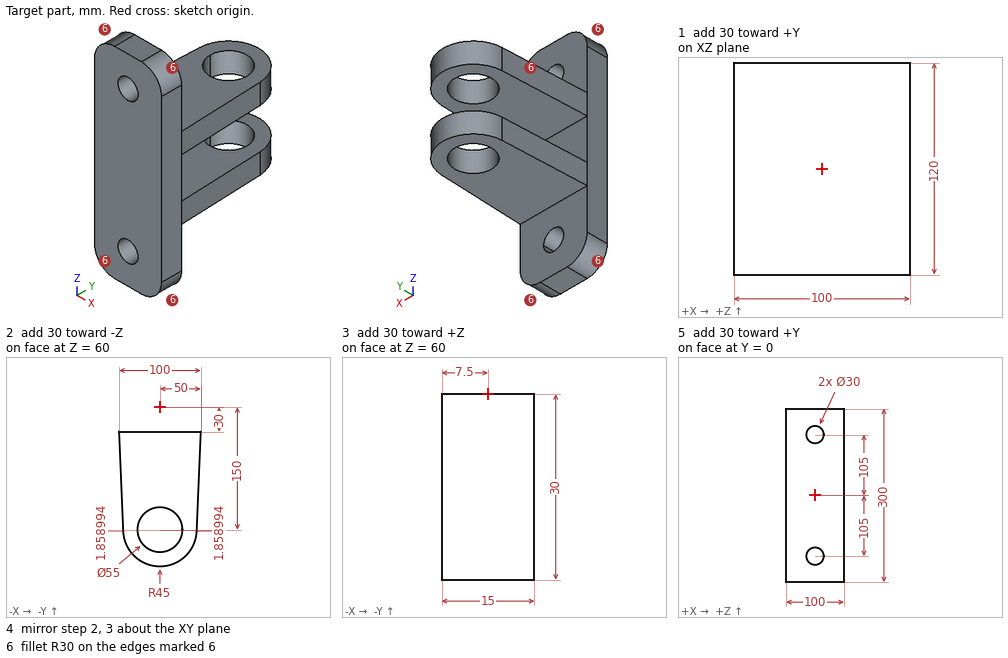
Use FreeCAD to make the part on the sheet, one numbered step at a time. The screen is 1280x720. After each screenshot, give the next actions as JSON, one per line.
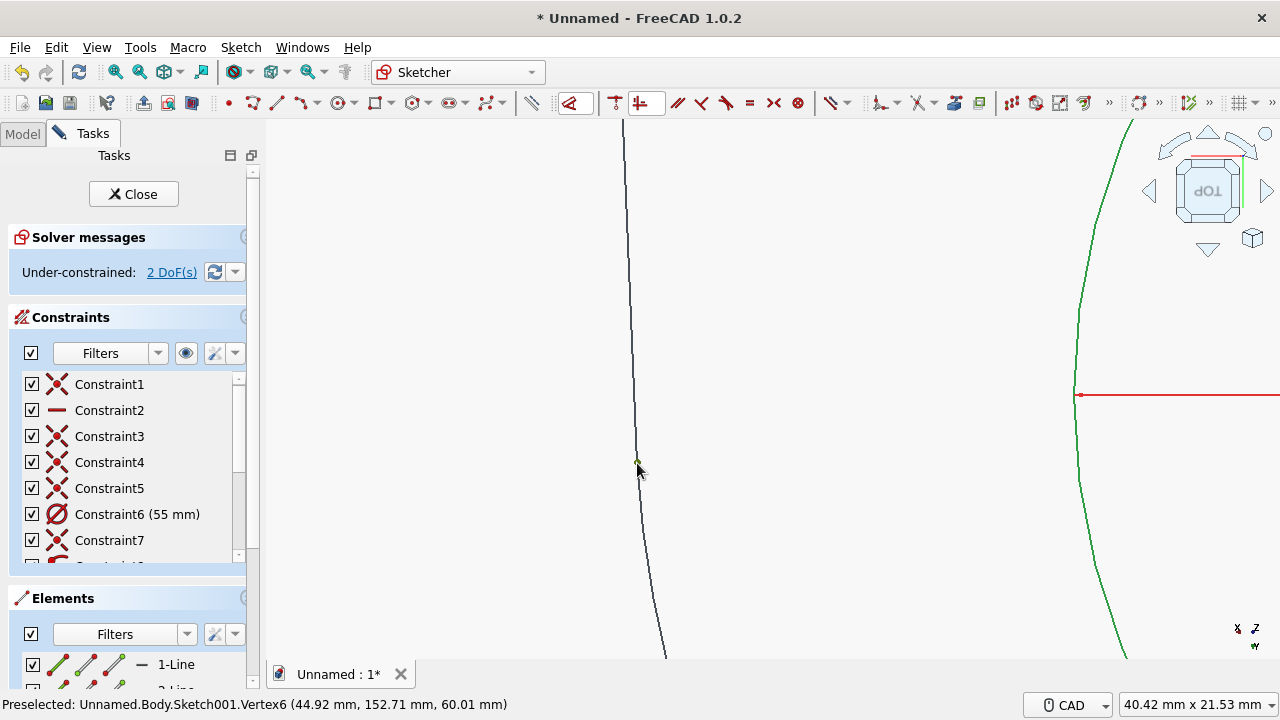
{"action": "scroll", "coordinate": [620, 494], "scroll_direction": "down", "scroll_amount": 13}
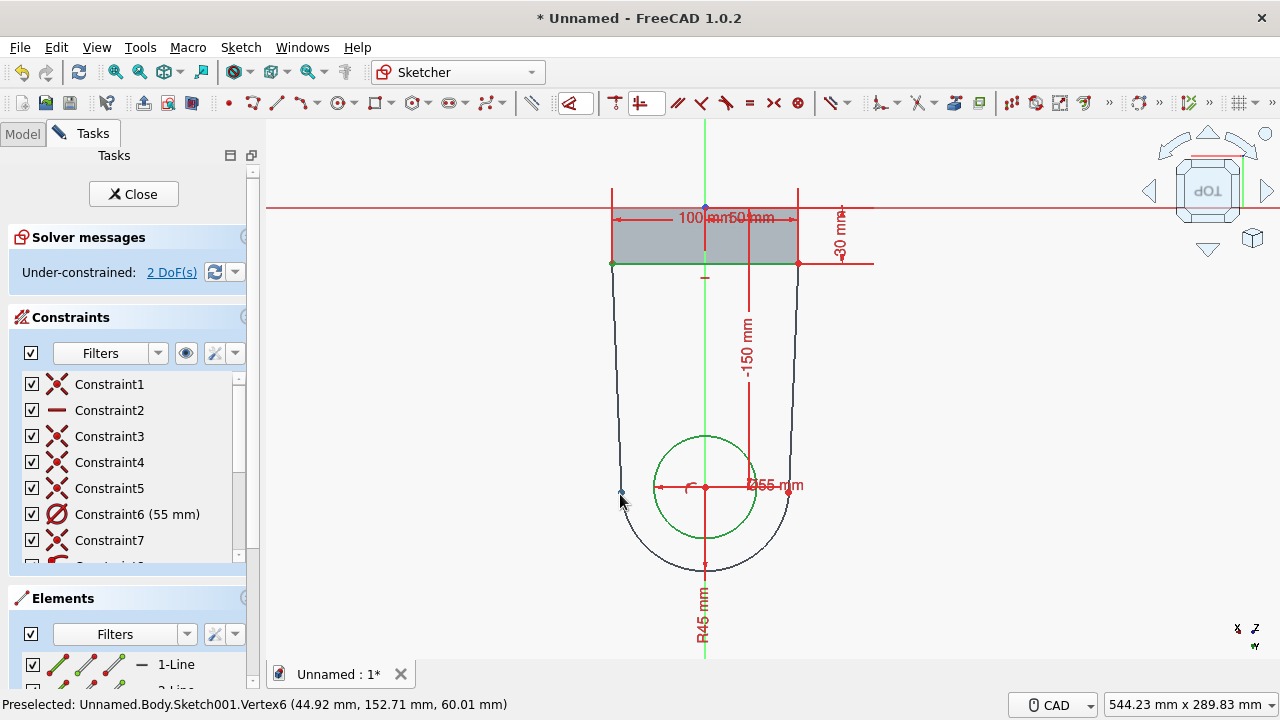
{"action": "scroll", "coordinate": [705, 487], "scroll_direction": "up", "scroll_amount": 13}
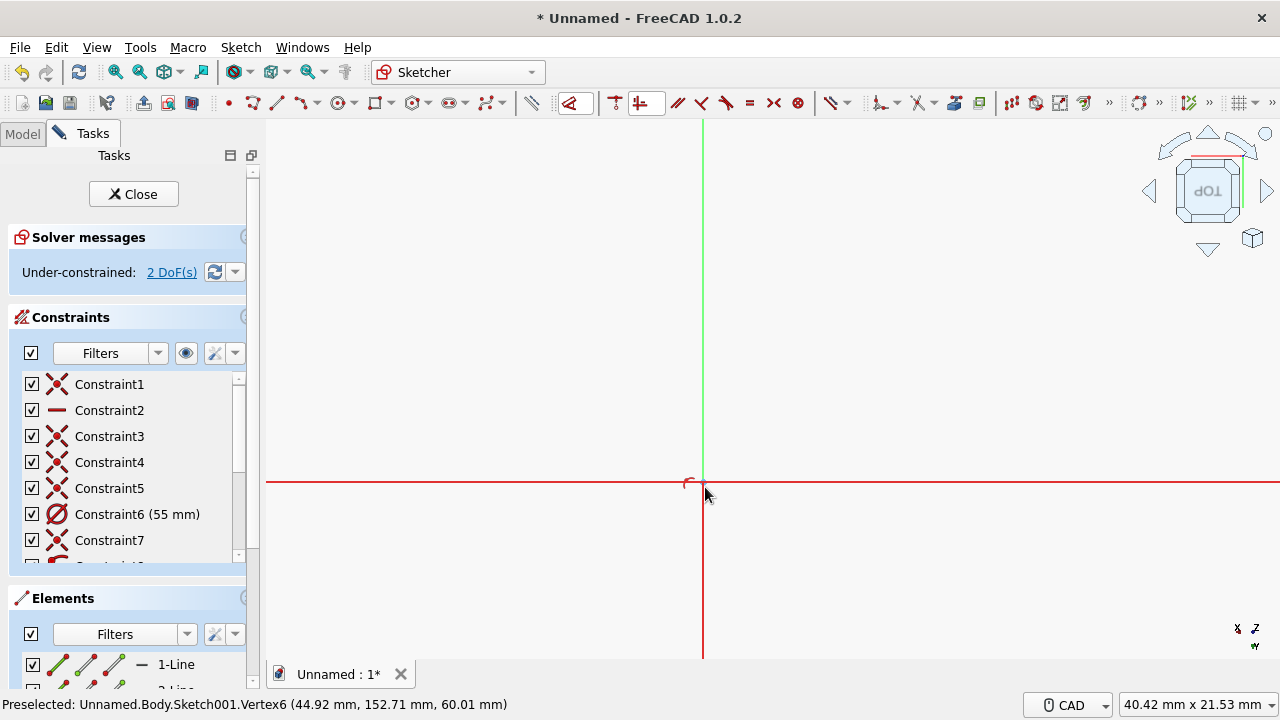
{"action": "left_click", "coordinate": [703, 482]}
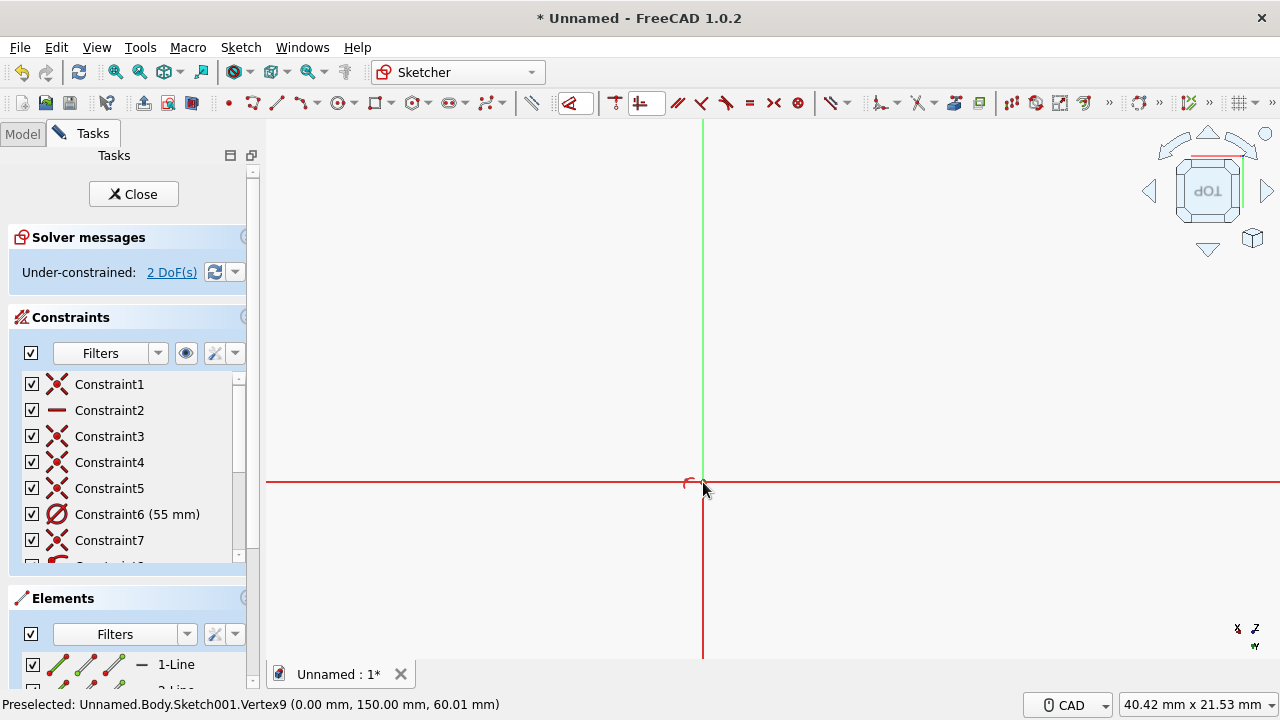
{"action": "key", "text": "i"}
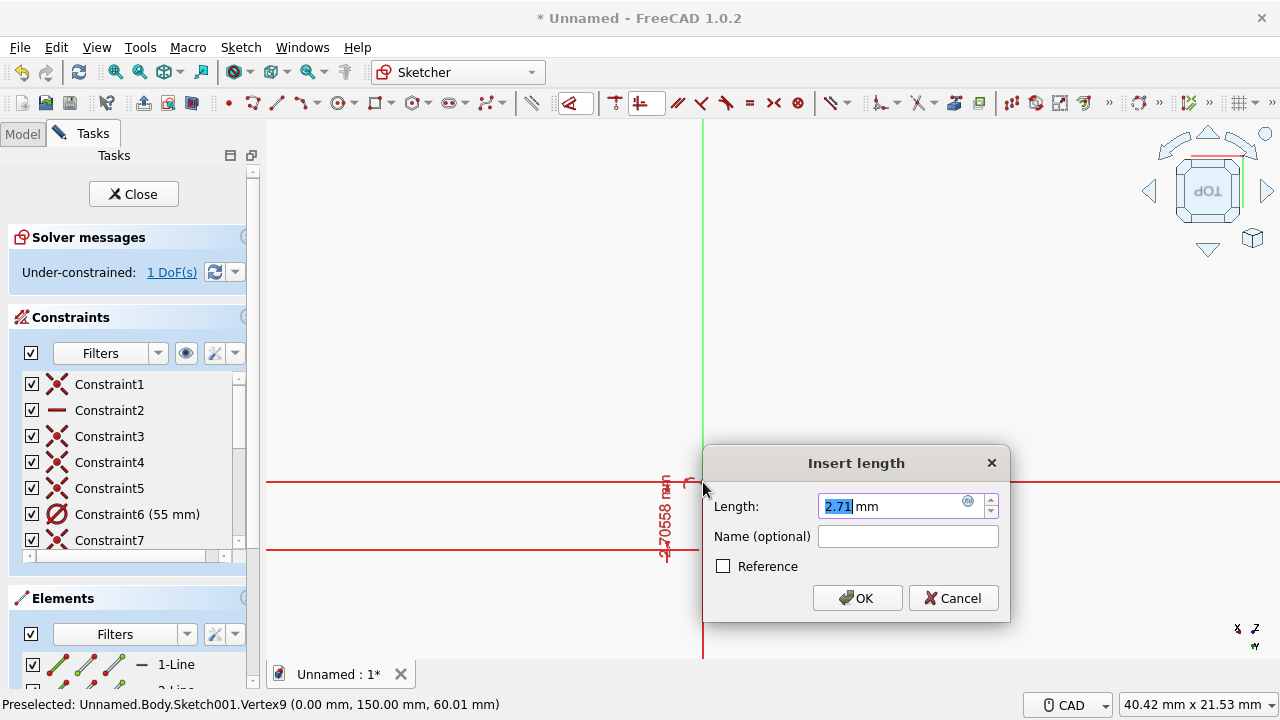
{"action": "type", "text": "1.858994"}
{"action": "key", "text": "Return"}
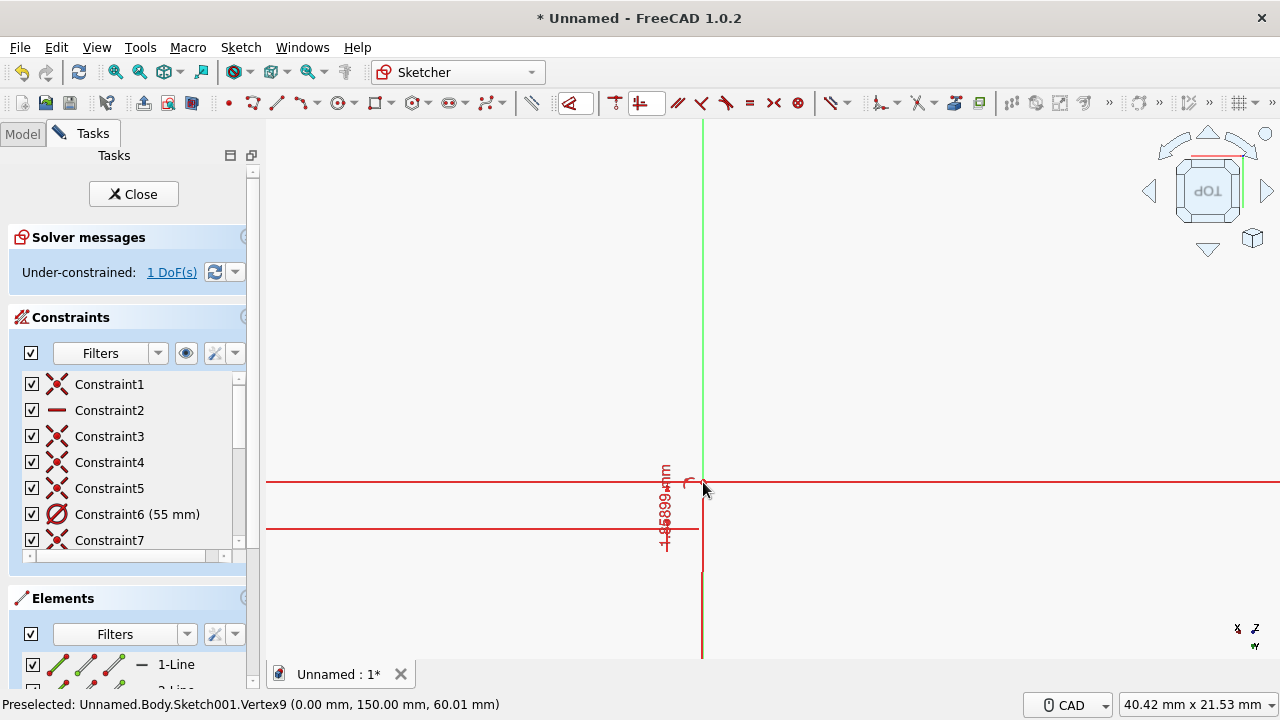
{"action": "scroll", "coordinate": [705, 487], "scroll_direction": "down", "scroll_amount": 13}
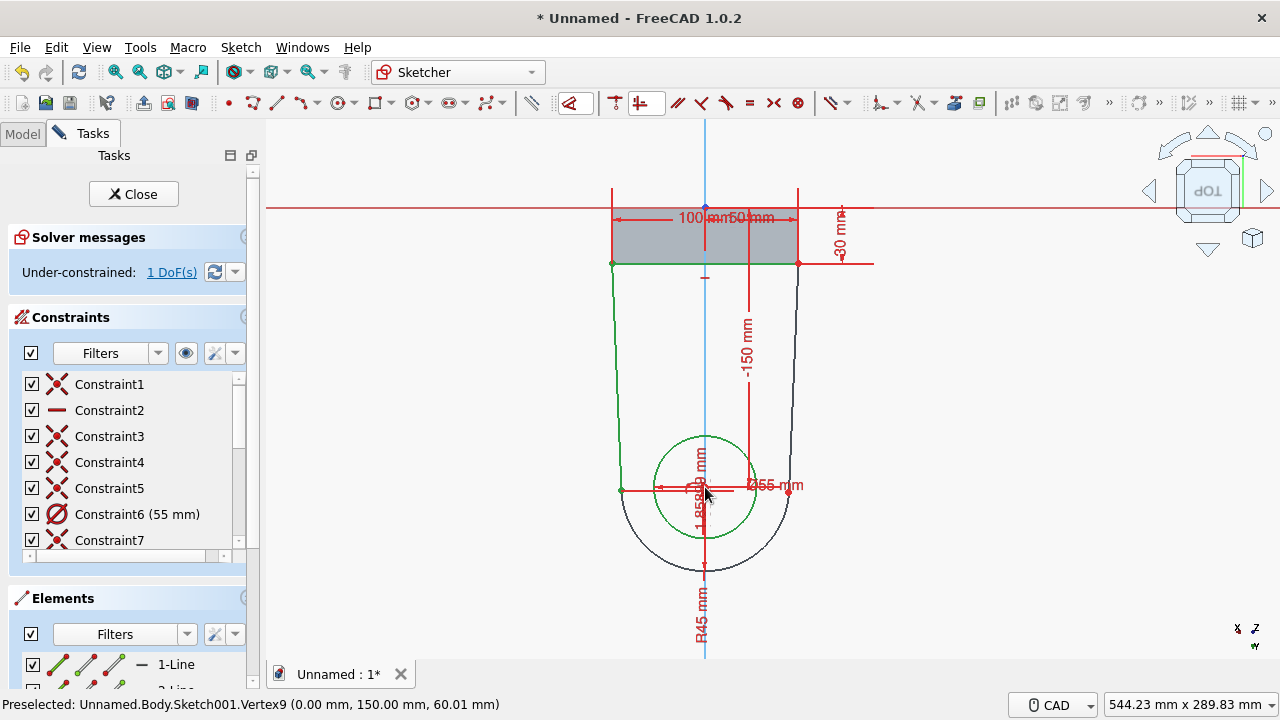
{"action": "scroll", "coordinate": [789, 492], "scroll_direction": "up", "scroll_amount": 13}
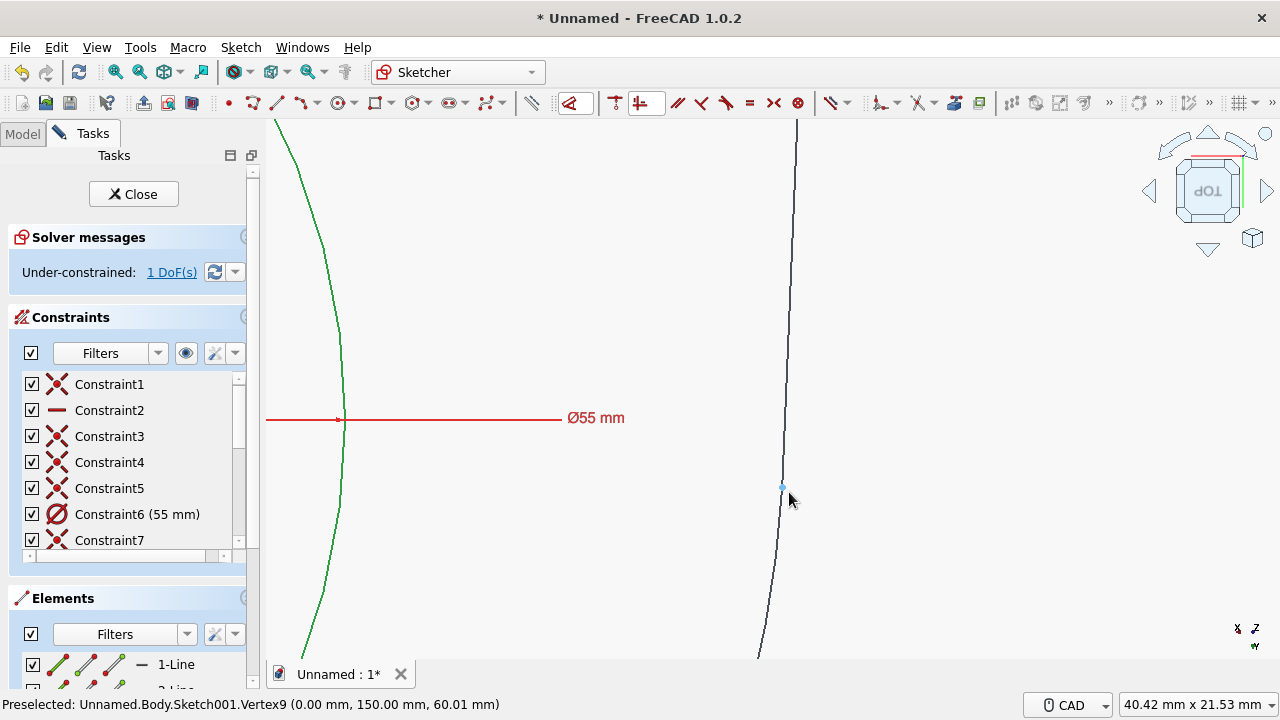
{"action": "left_click", "coordinate": [782, 488]}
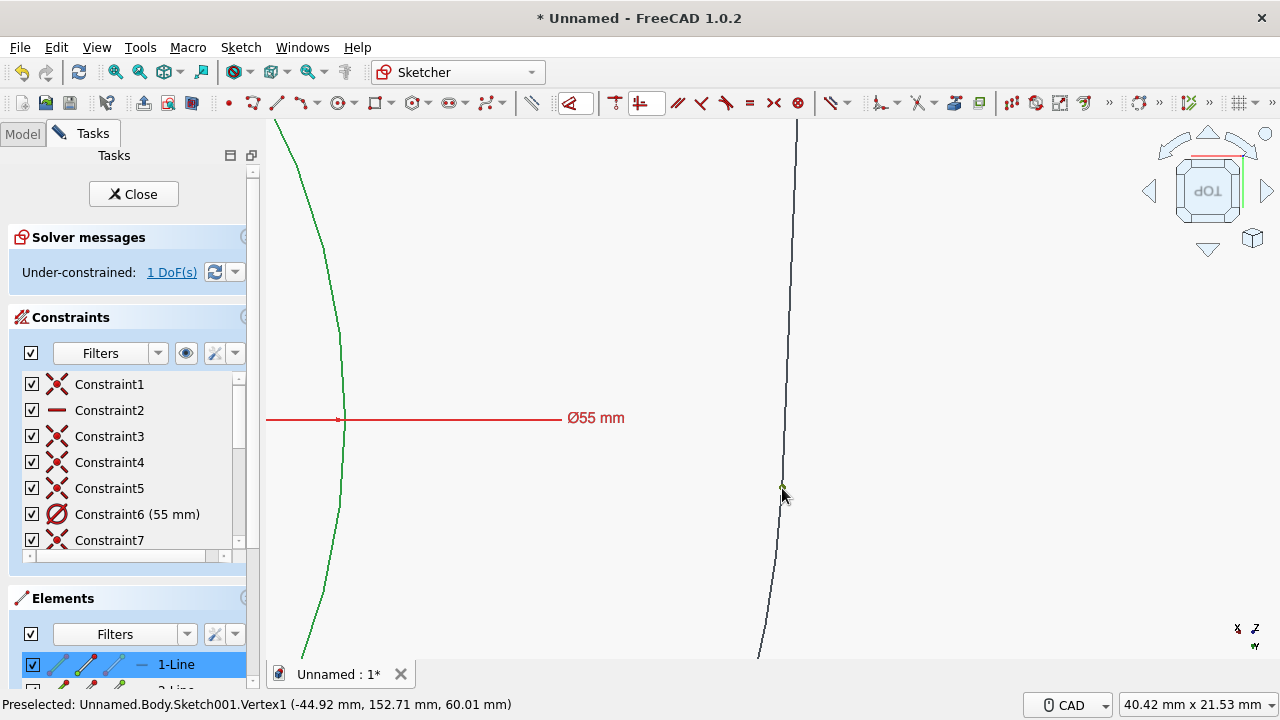
{"action": "scroll", "coordinate": [789, 492], "scroll_direction": "down", "scroll_amount": 13}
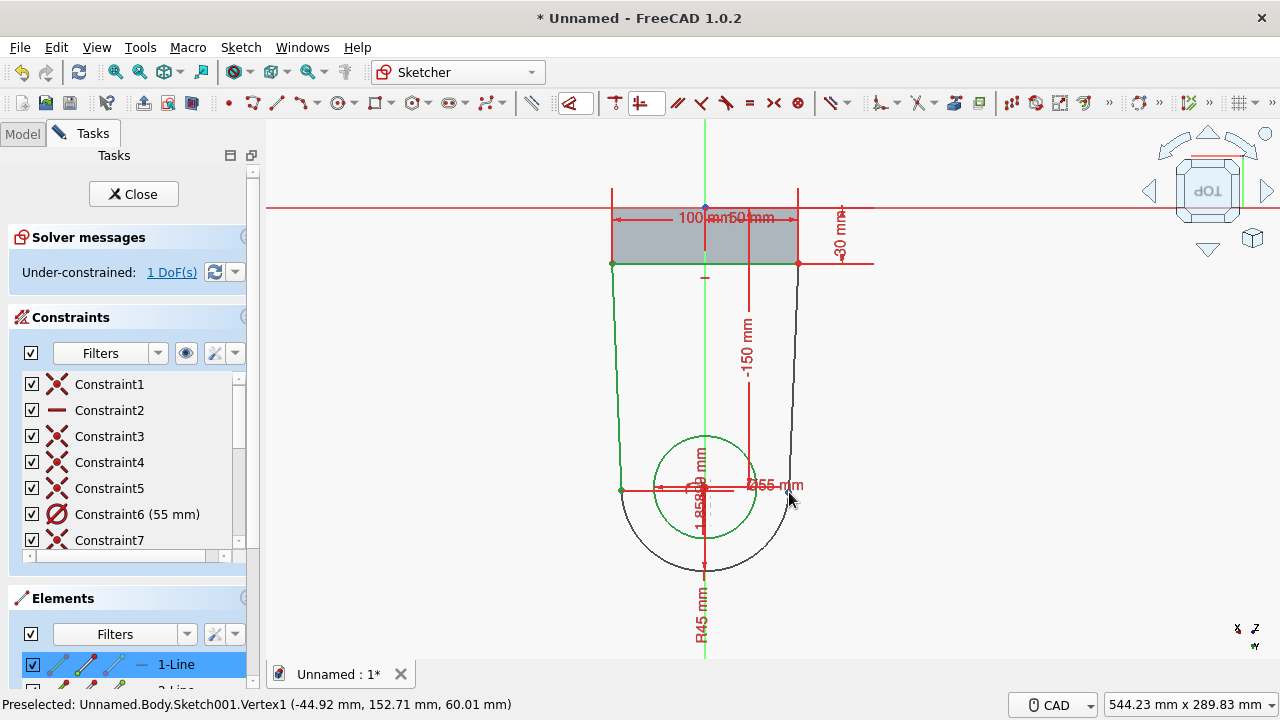
{"action": "scroll", "coordinate": [705, 487], "scroll_direction": "up", "scroll_amount": 13}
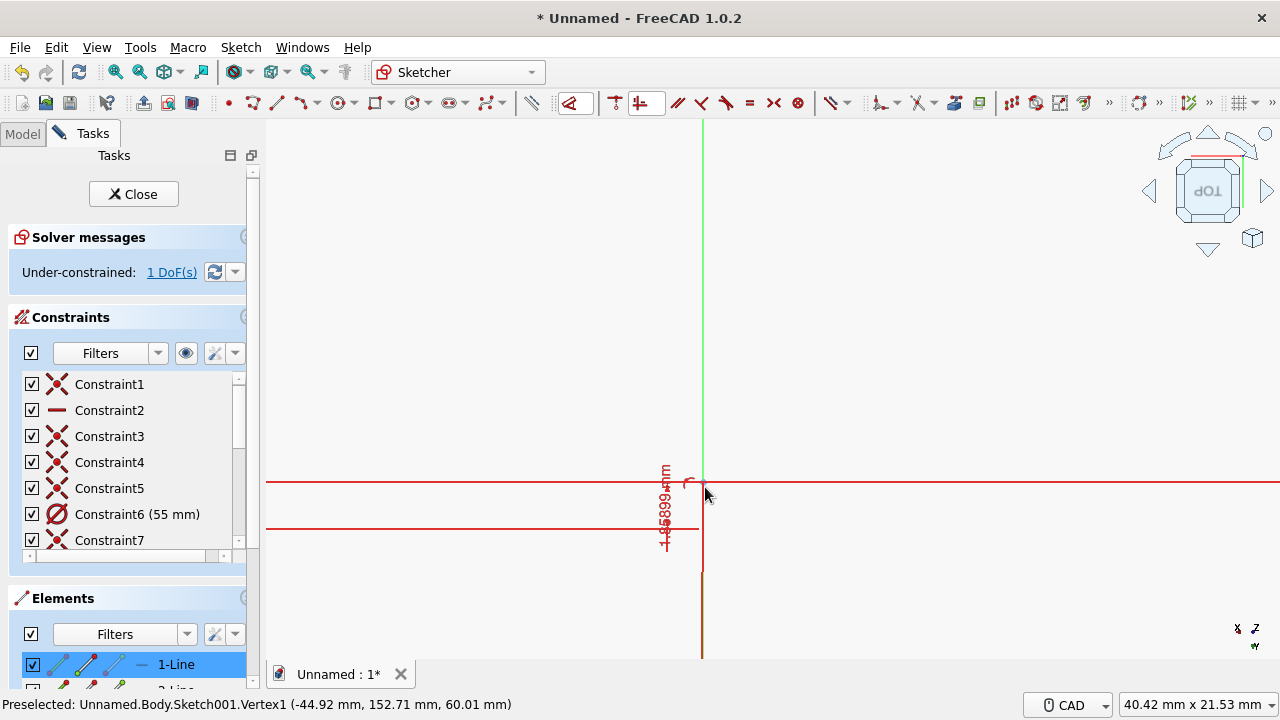
{"action": "left_click", "coordinate": [703, 482]}